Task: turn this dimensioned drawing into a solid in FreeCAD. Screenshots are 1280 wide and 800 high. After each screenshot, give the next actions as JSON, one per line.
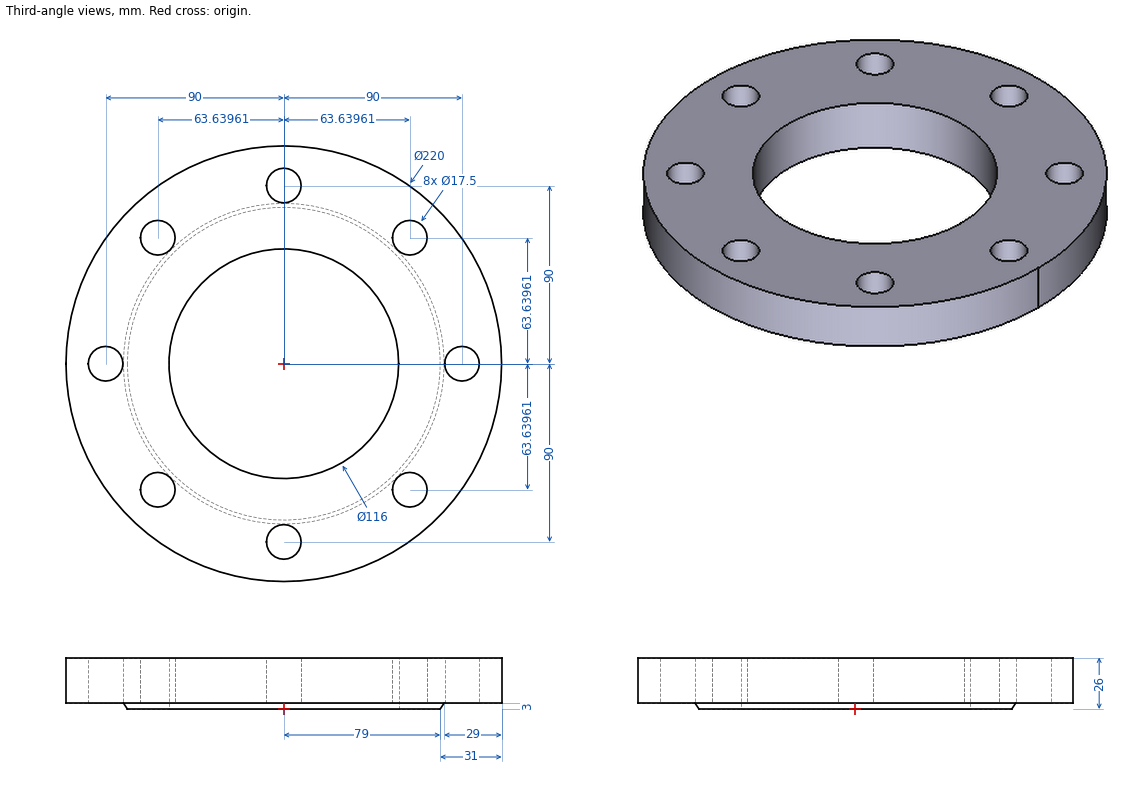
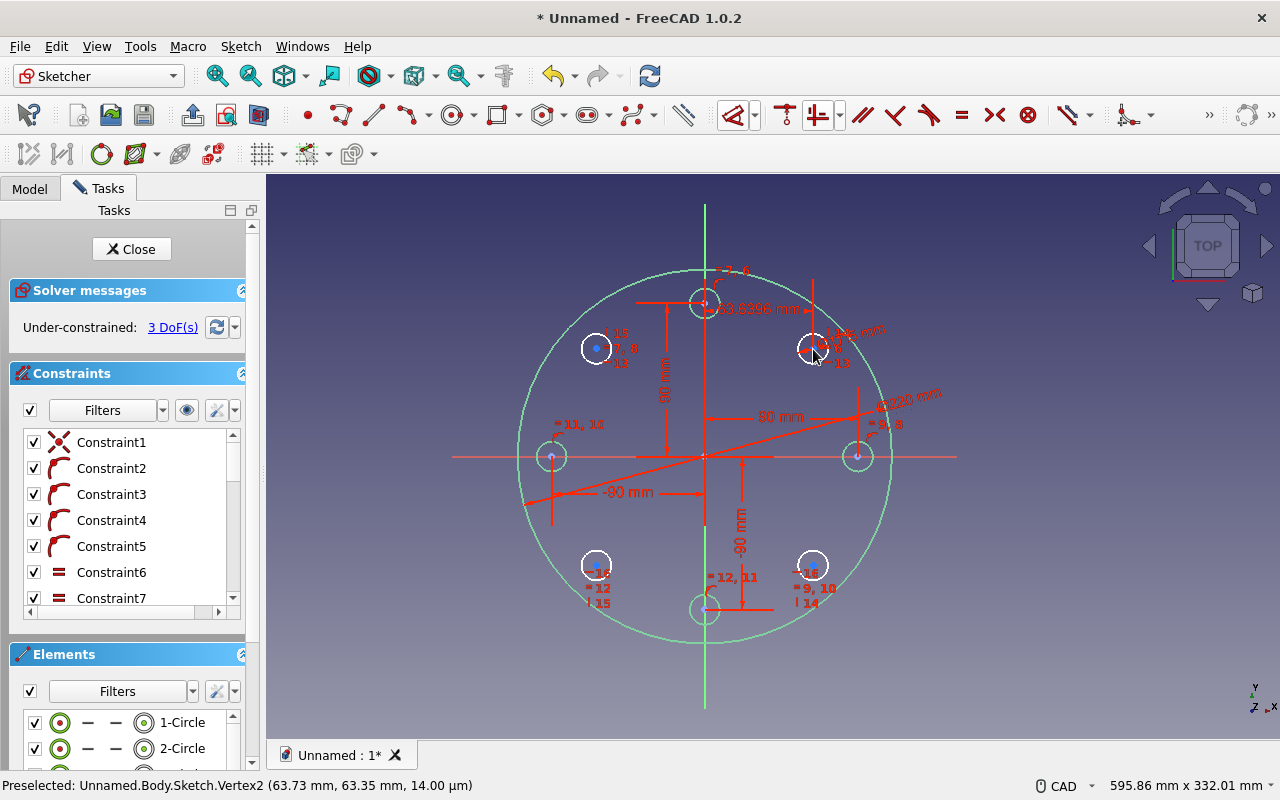
{"action": "left_click", "coordinate": [813, 349]}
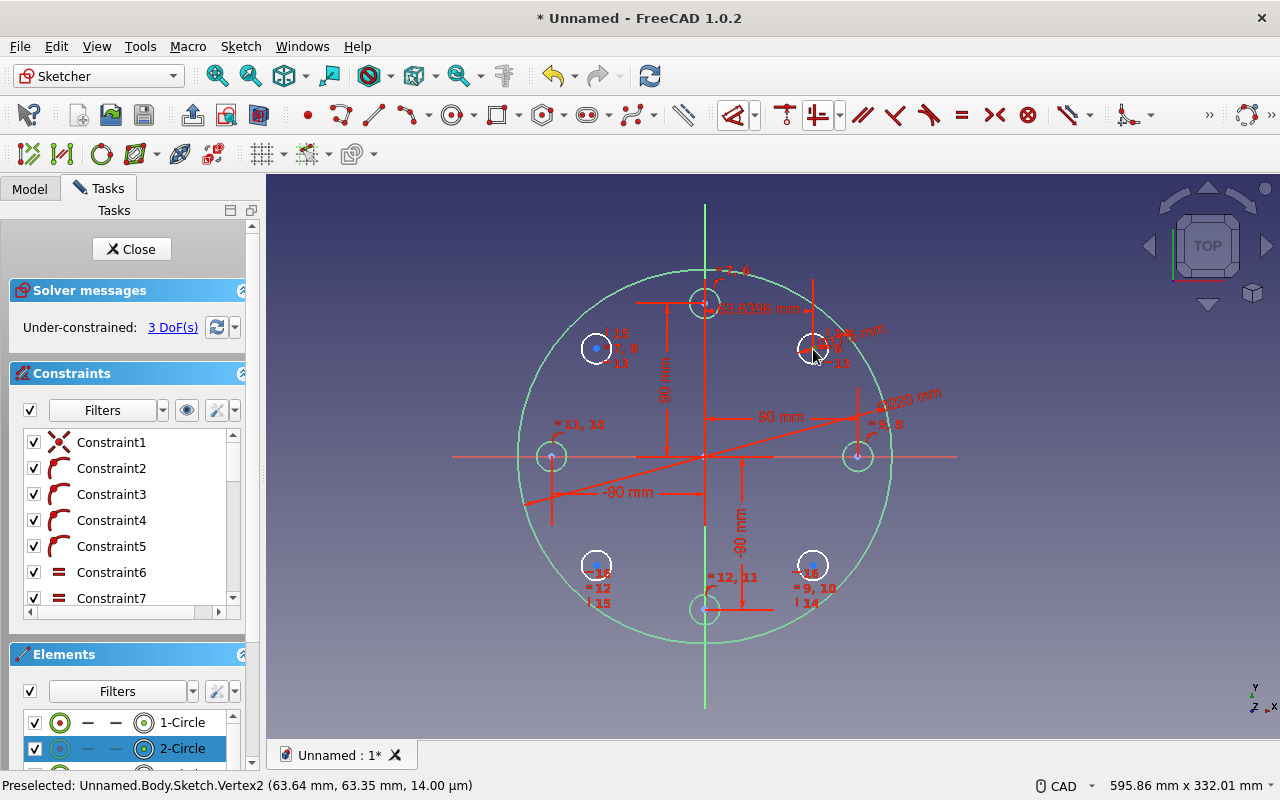
{"action": "key", "text": "i"}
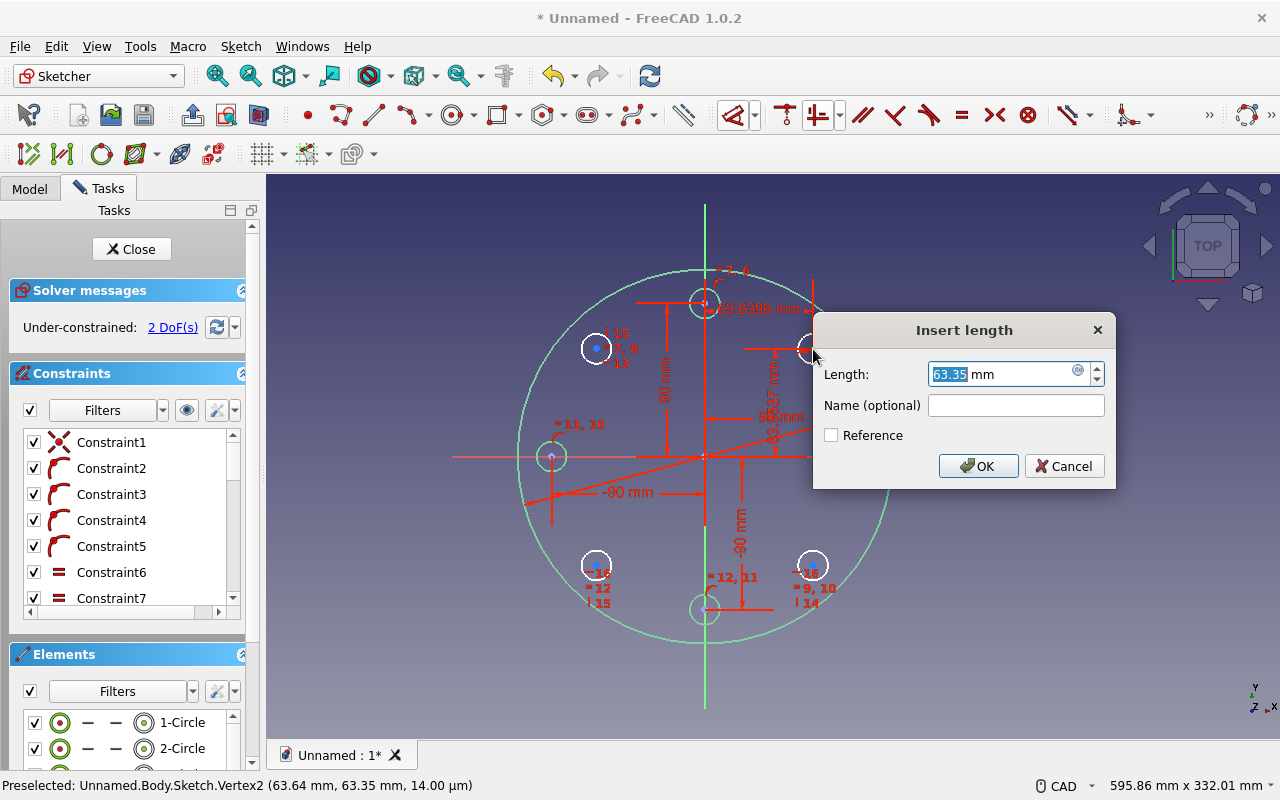
{"action": "type", "text": "63.63961"}
{"action": "key", "text": "Return"}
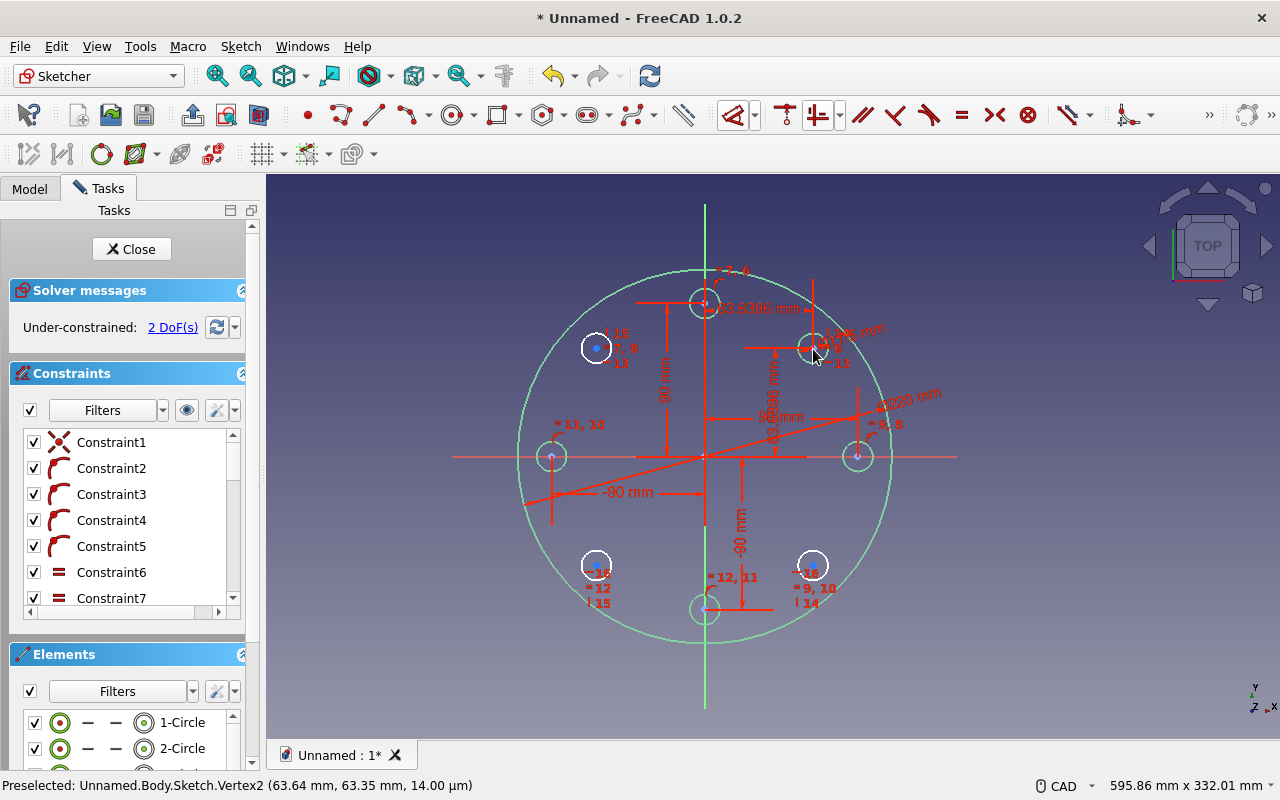
{"action": "left_click", "coordinate": [596, 348]}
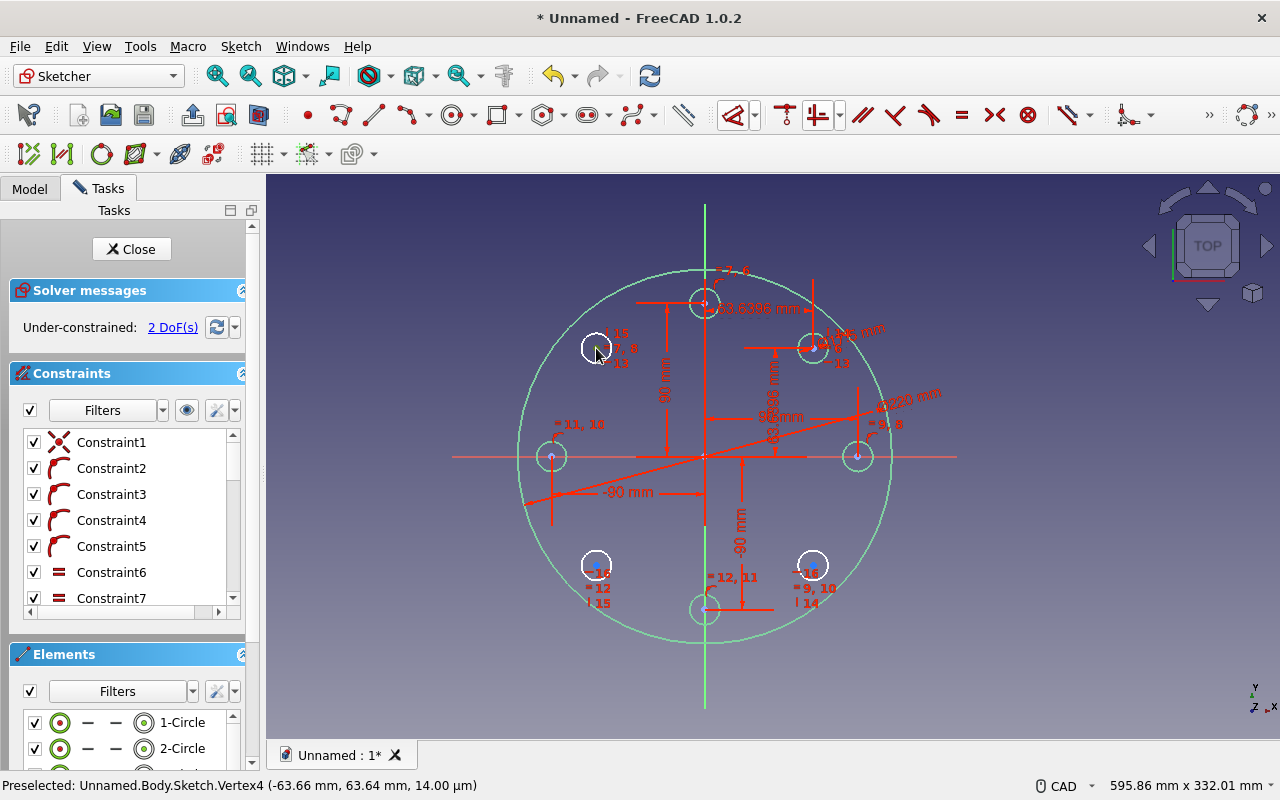
{"action": "key", "text": "l"}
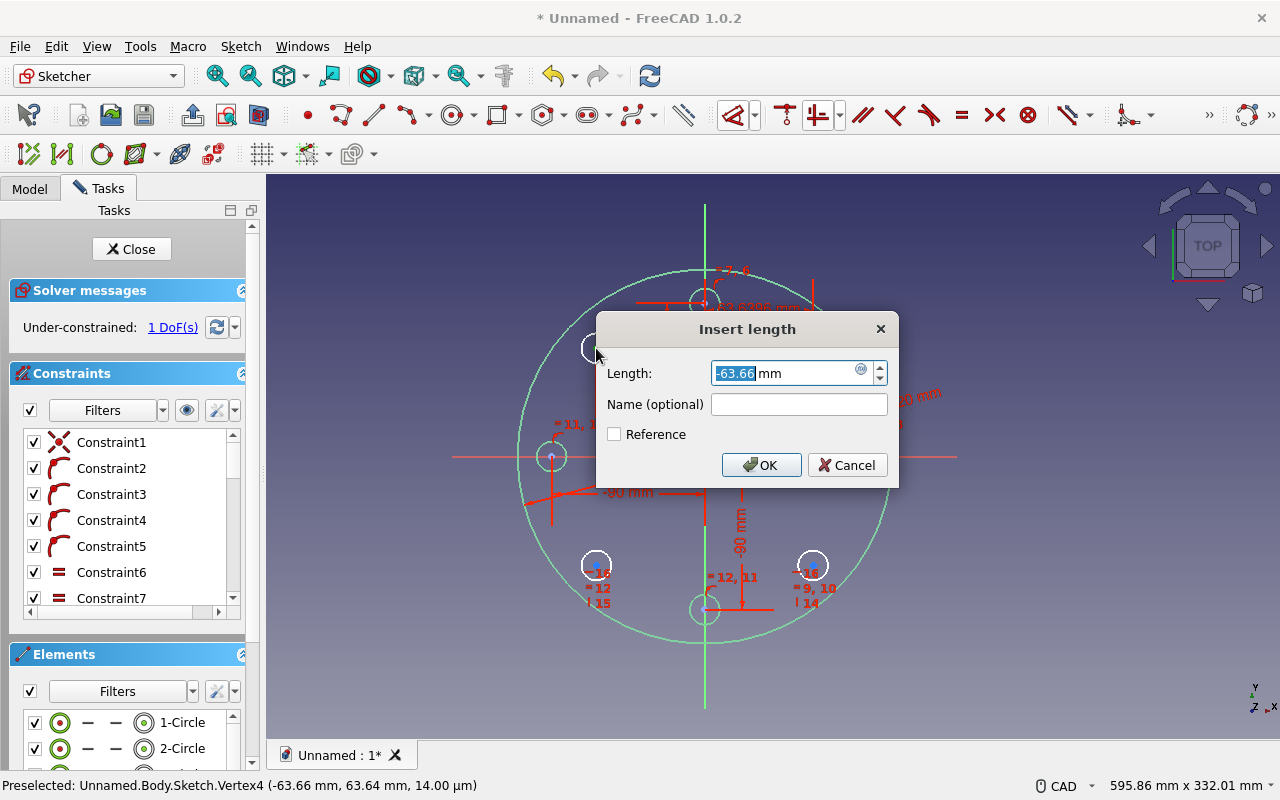
{"action": "type", "text": "-63.63961"}
{"action": "key", "text": "Return"}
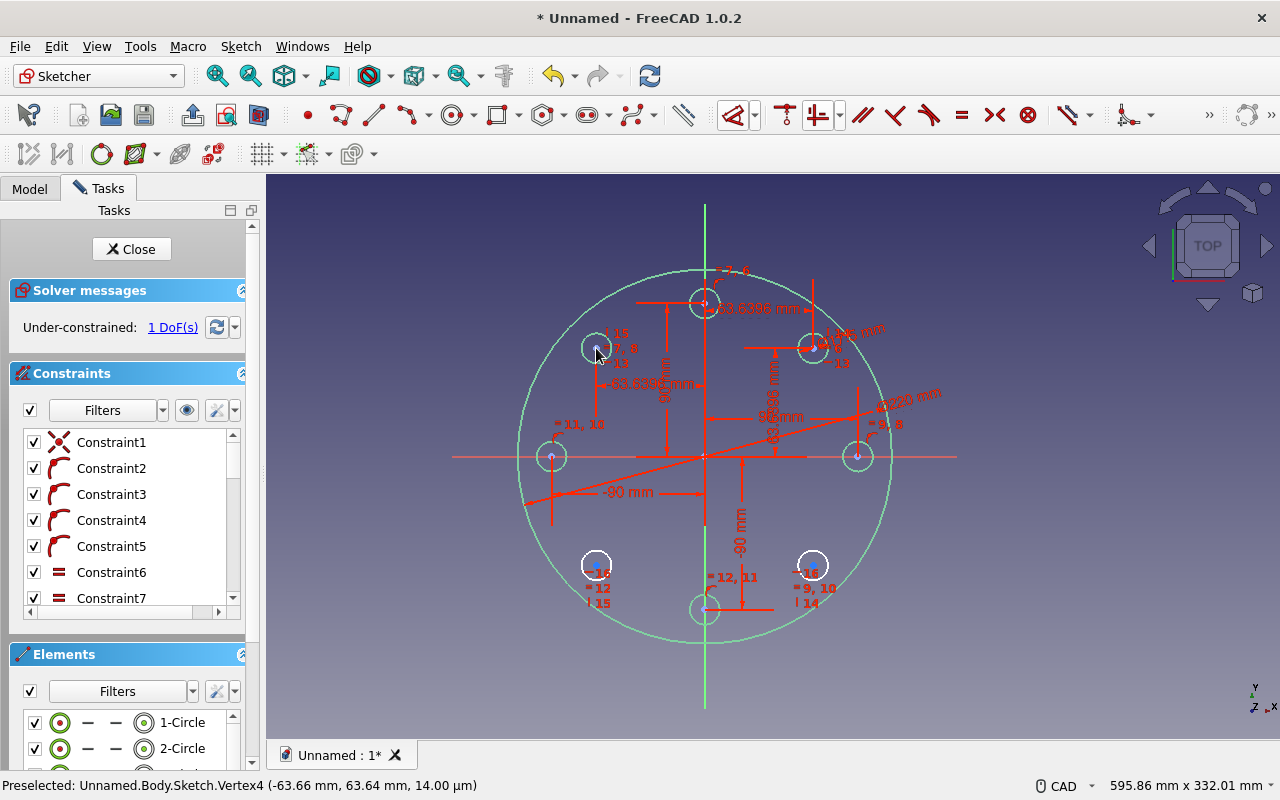
{"action": "left_click", "coordinate": [813, 565]}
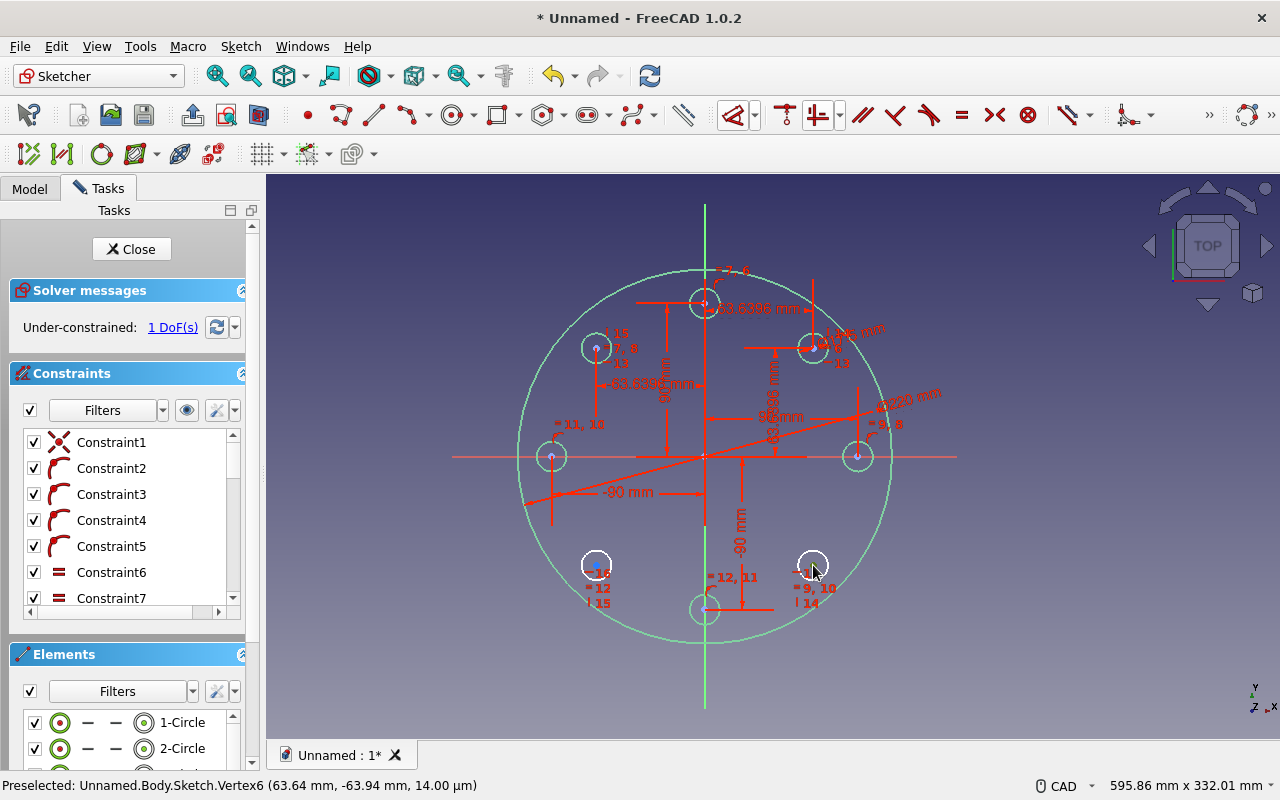
{"action": "key", "text": "i"}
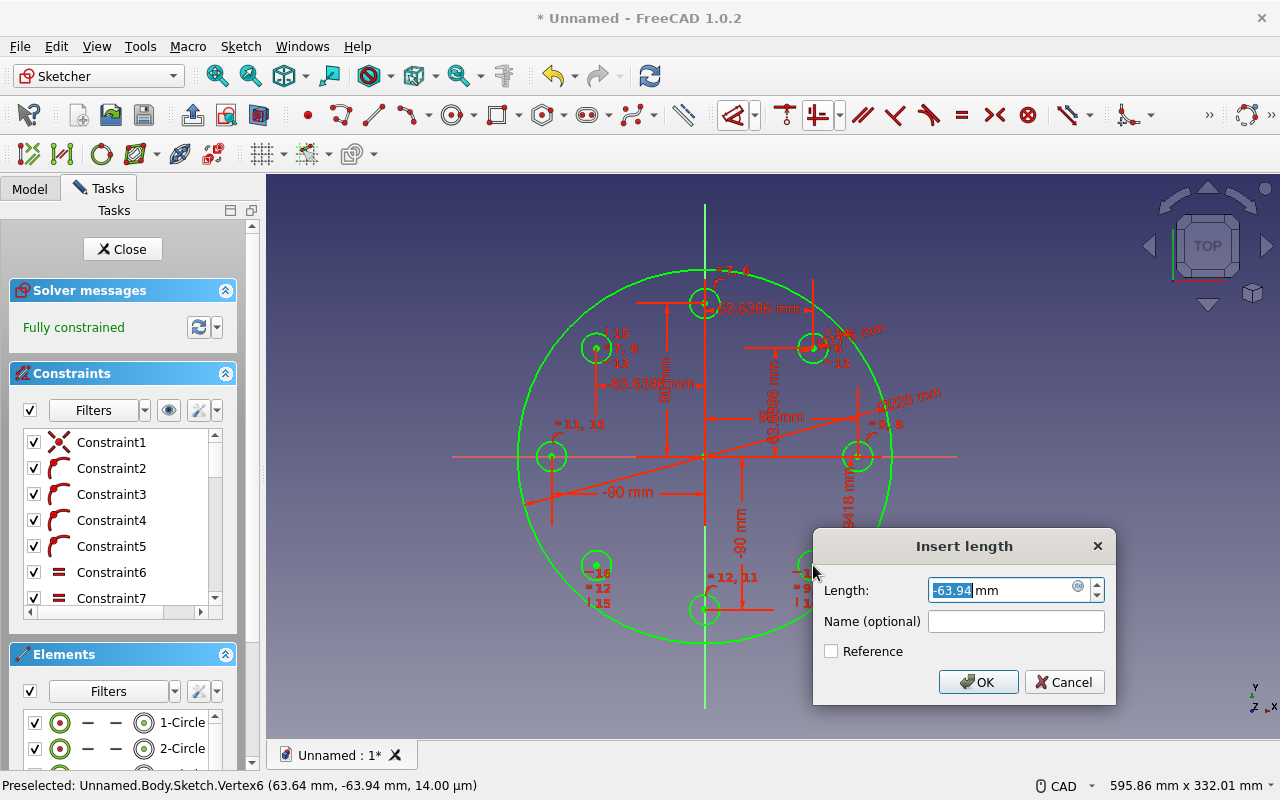
{"action": "type", "text": "-63.63961"}
{"action": "key", "text": "Return"}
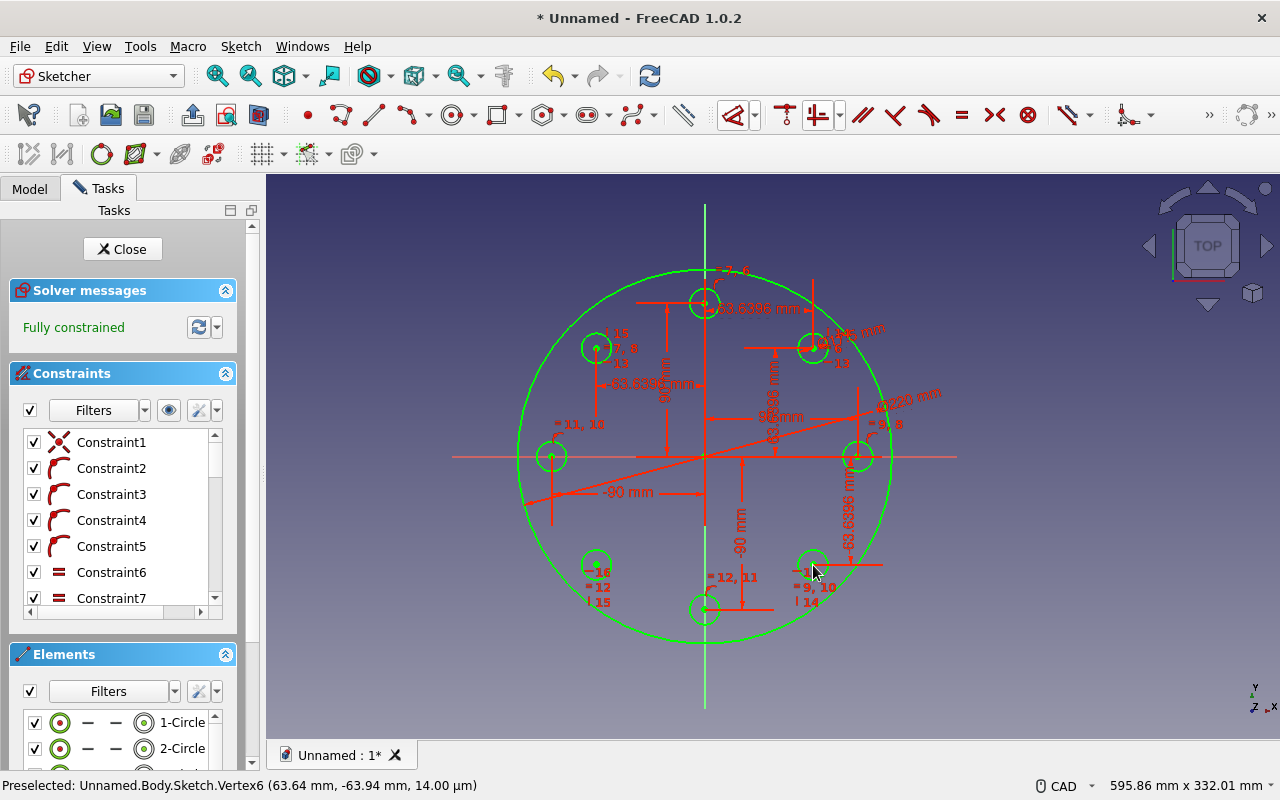
{"action": "left_click", "coordinate": [123, 249]}